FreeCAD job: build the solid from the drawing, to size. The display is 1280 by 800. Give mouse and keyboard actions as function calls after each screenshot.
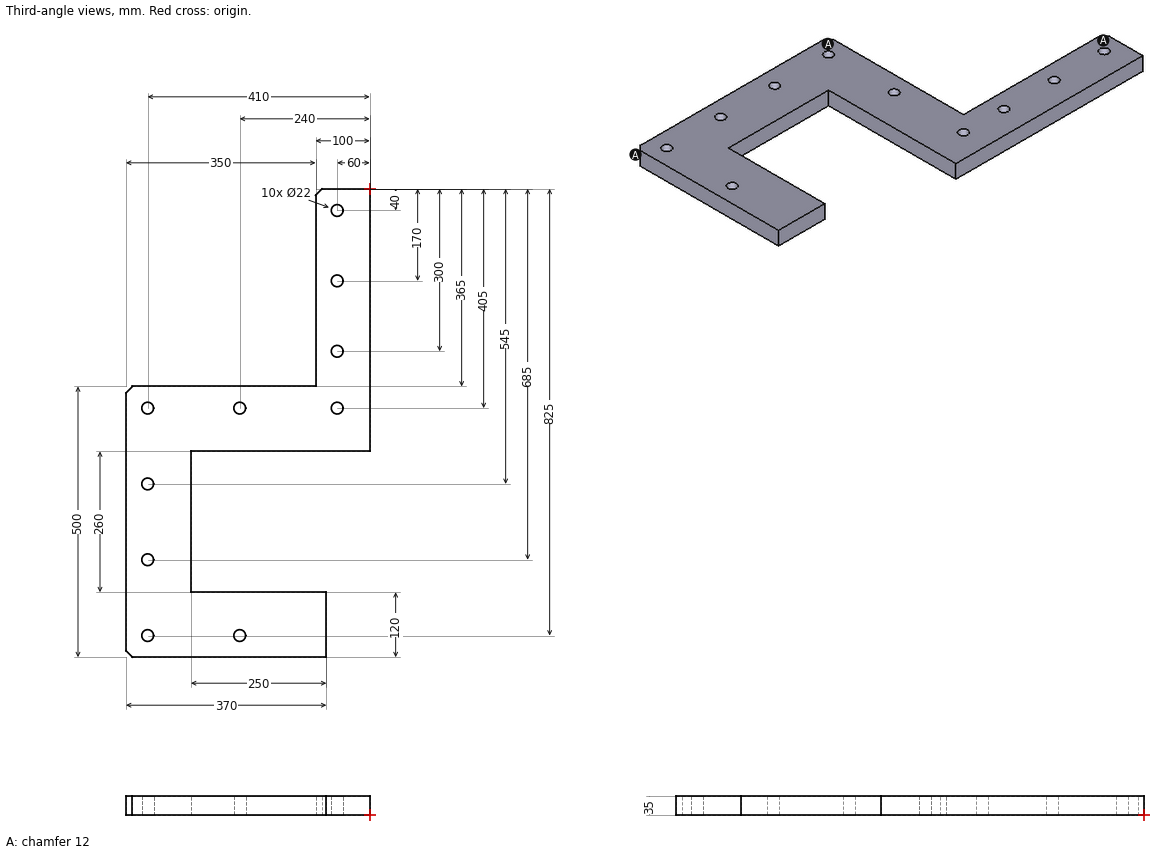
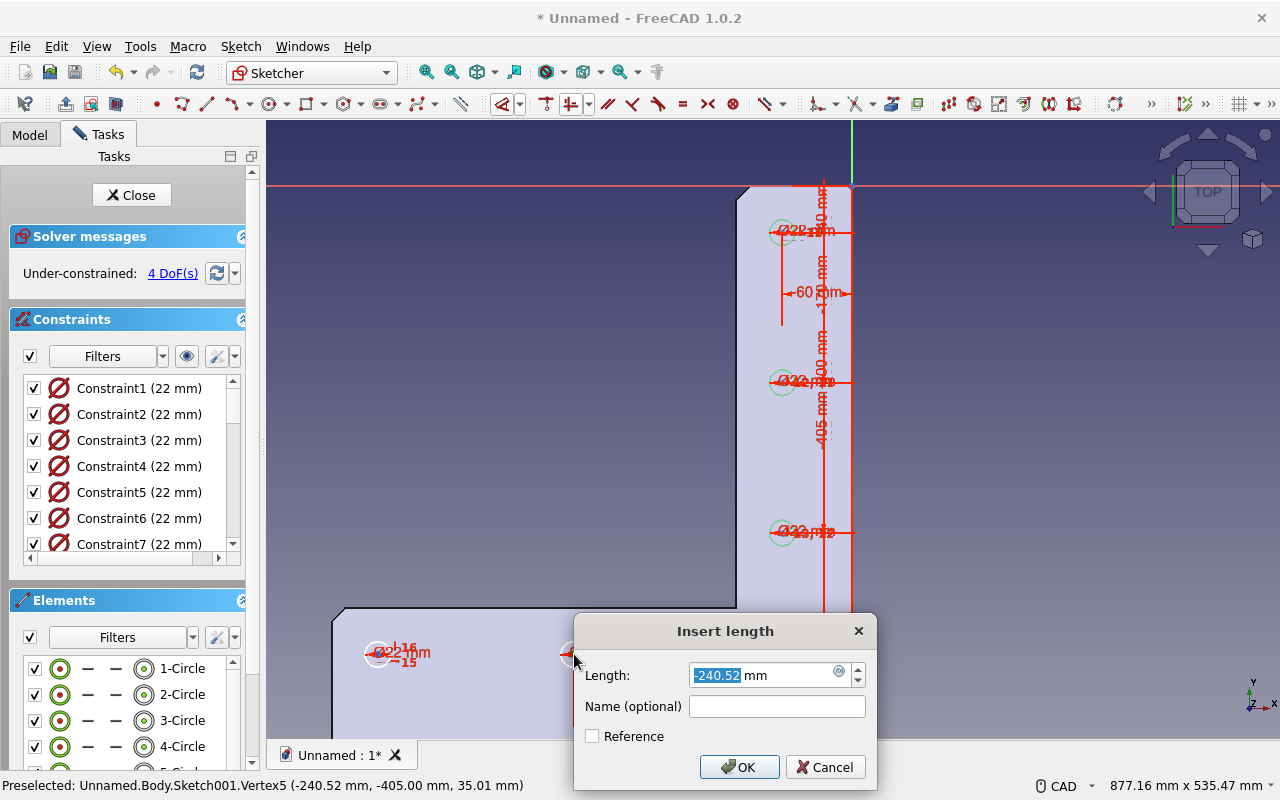
text(-240)
key(Return)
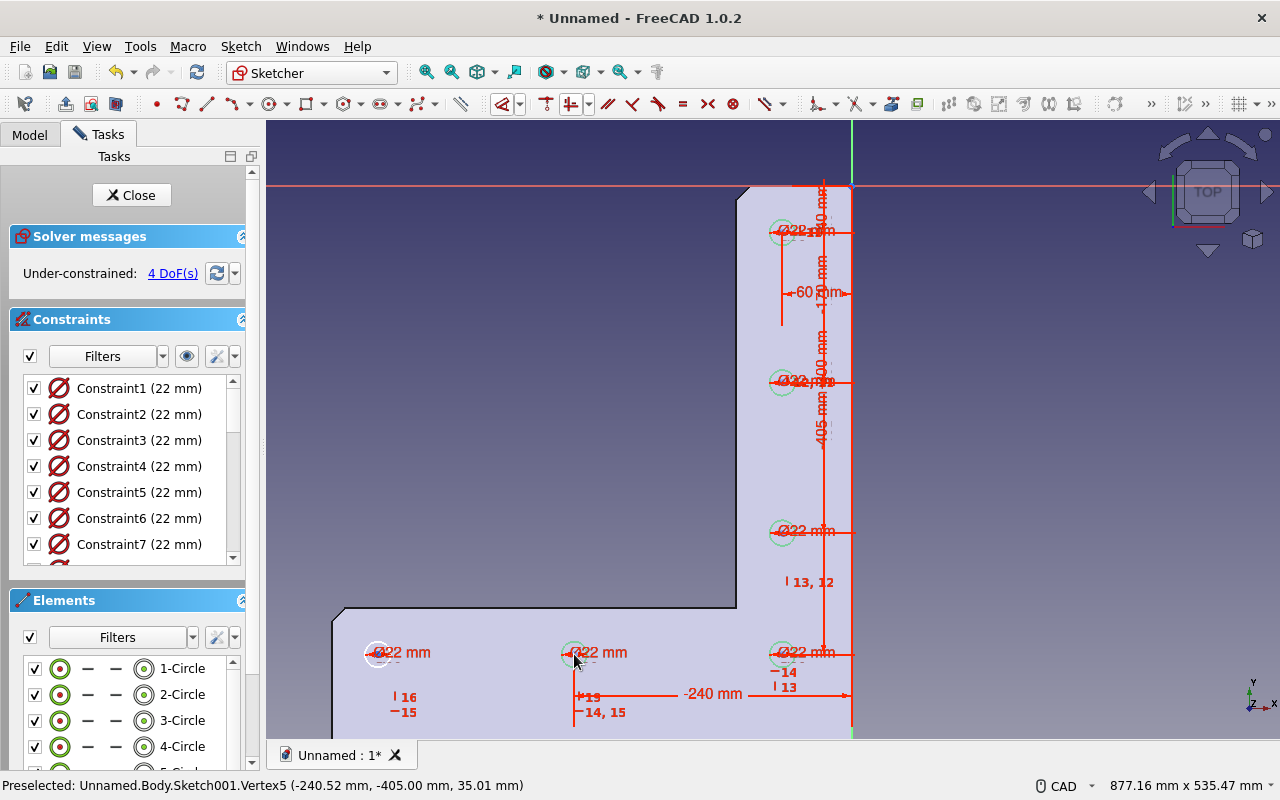
click(378, 654)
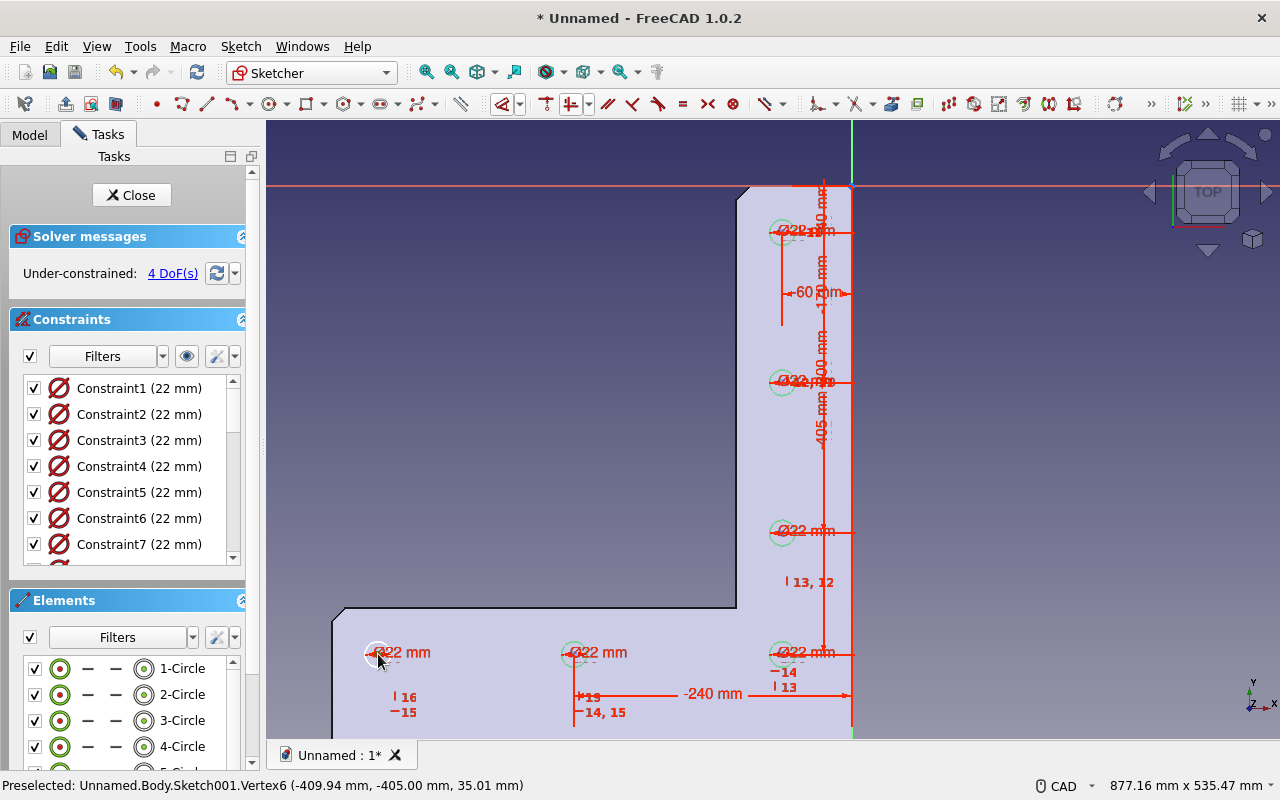
key(l)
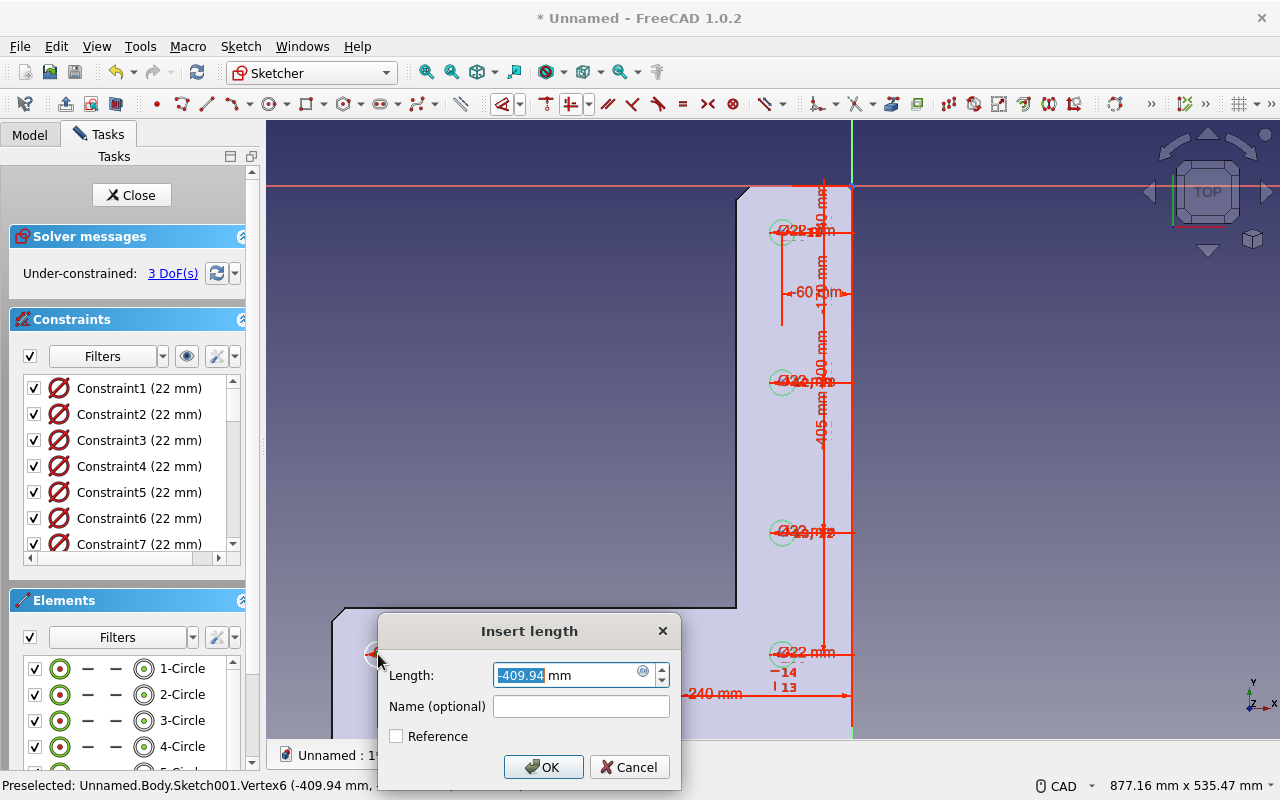
text(-410)
key(Return)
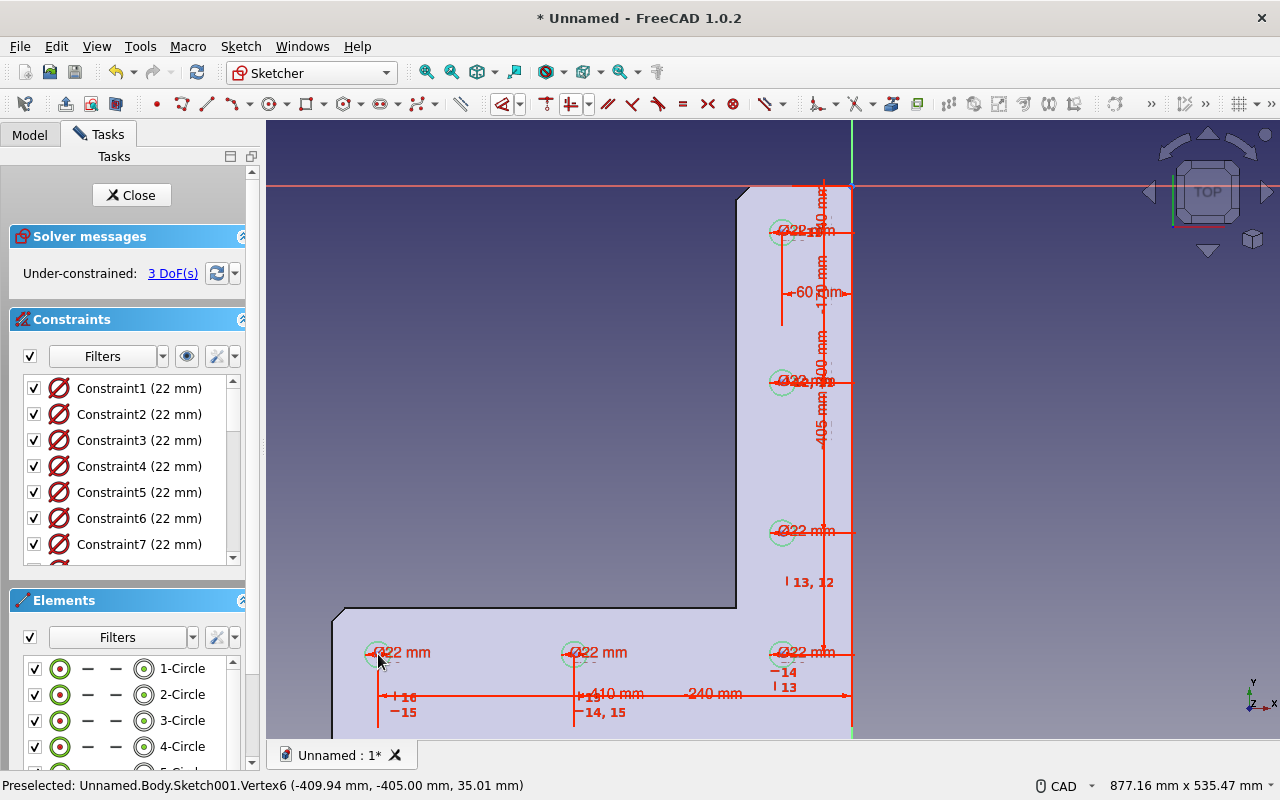
scroll(783, 234, down, 4)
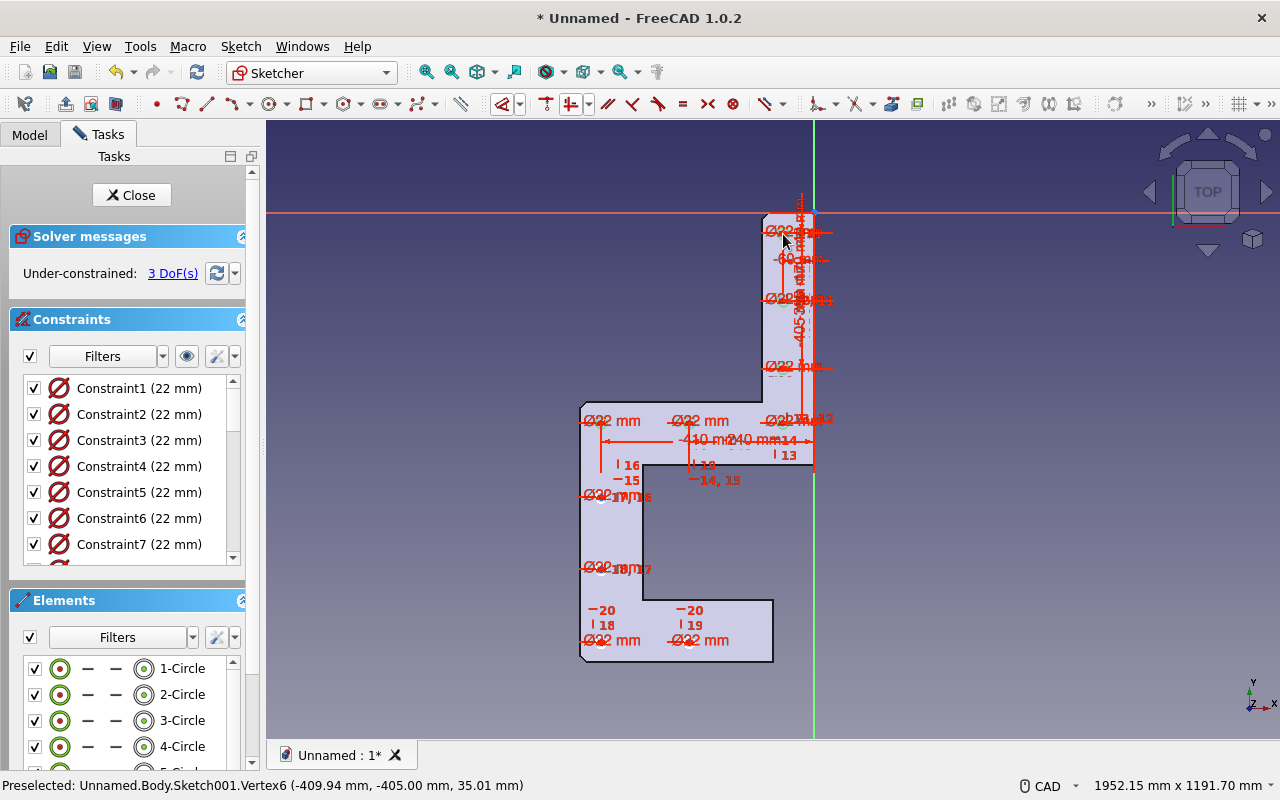
click(601, 497)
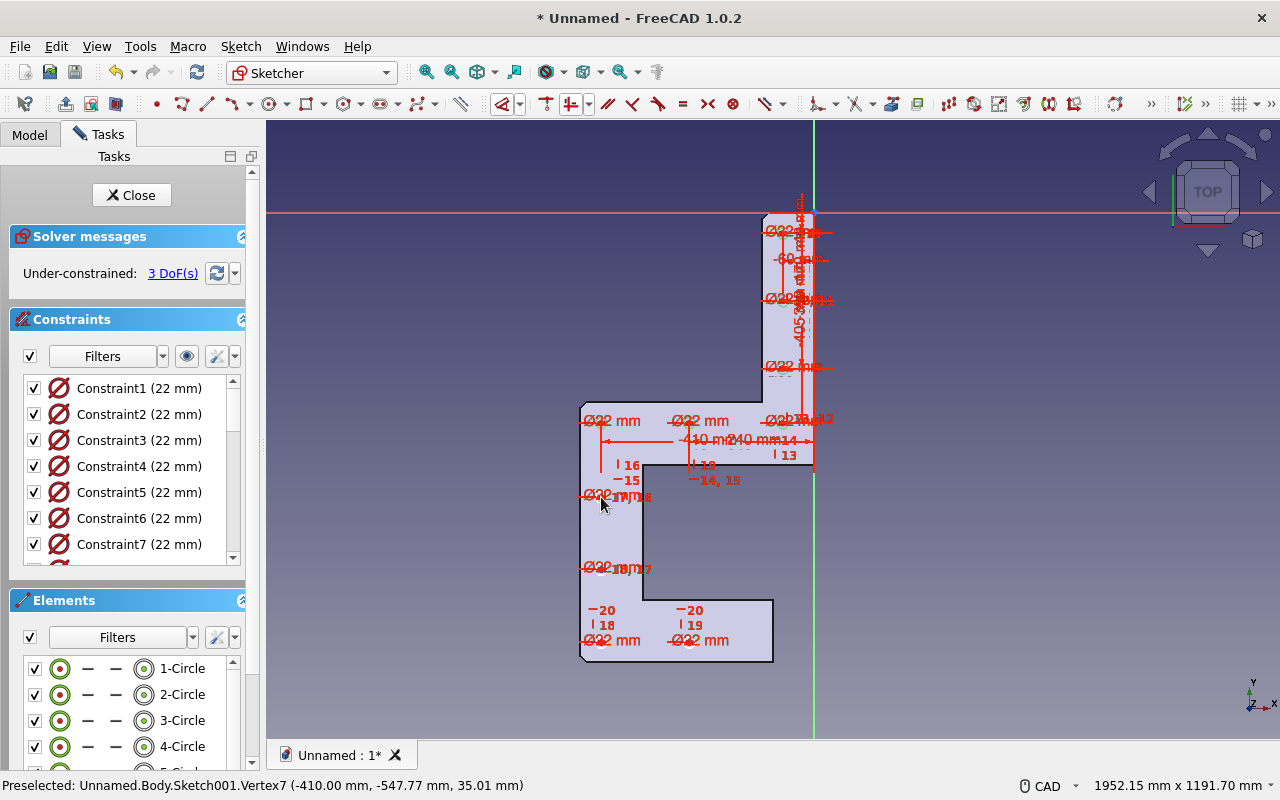
click(520, 104)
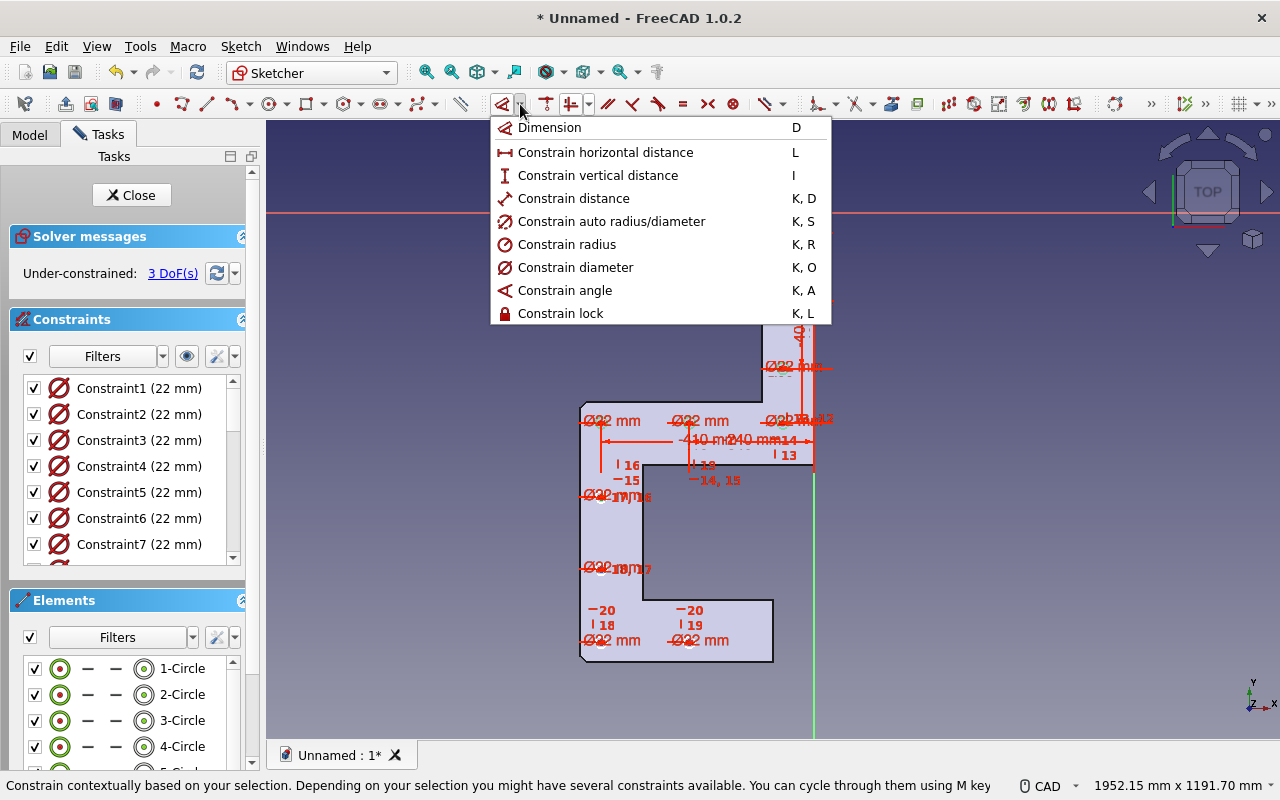
click(661, 176)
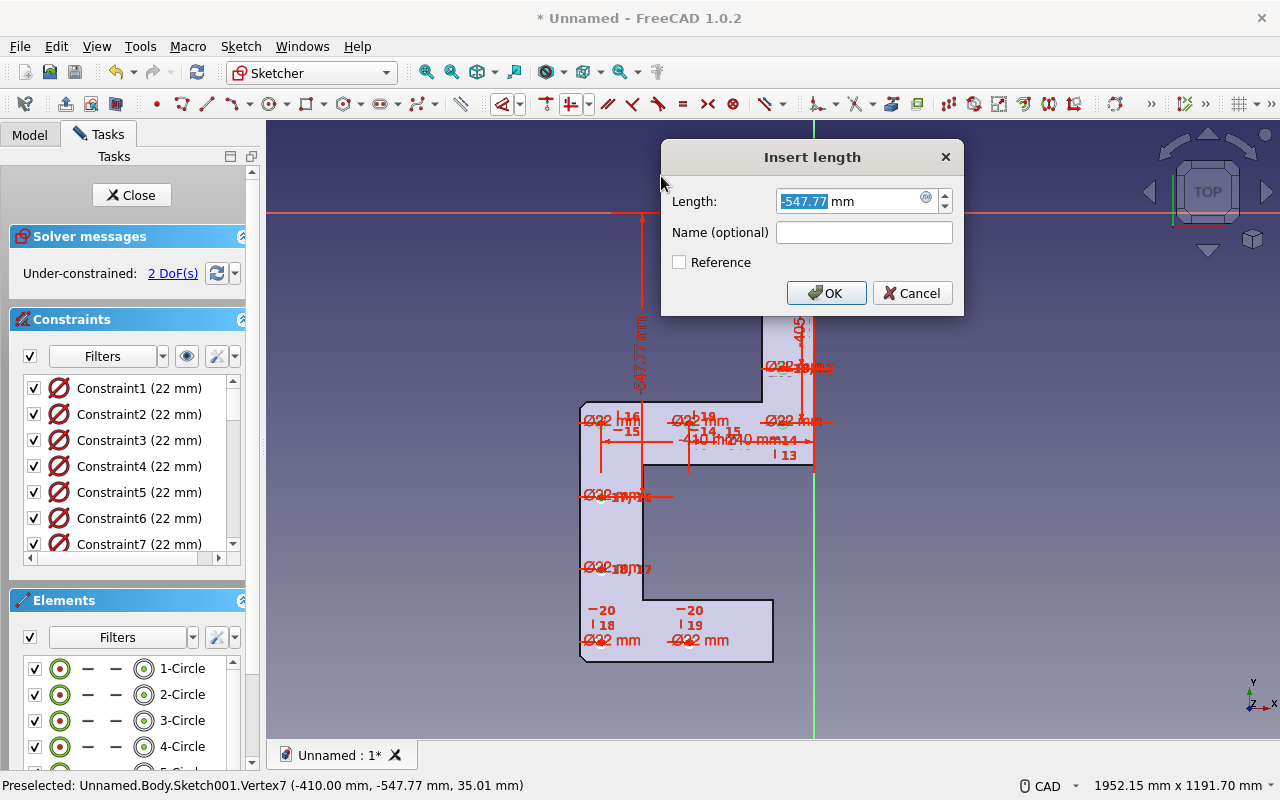
text(-545)
key(Return)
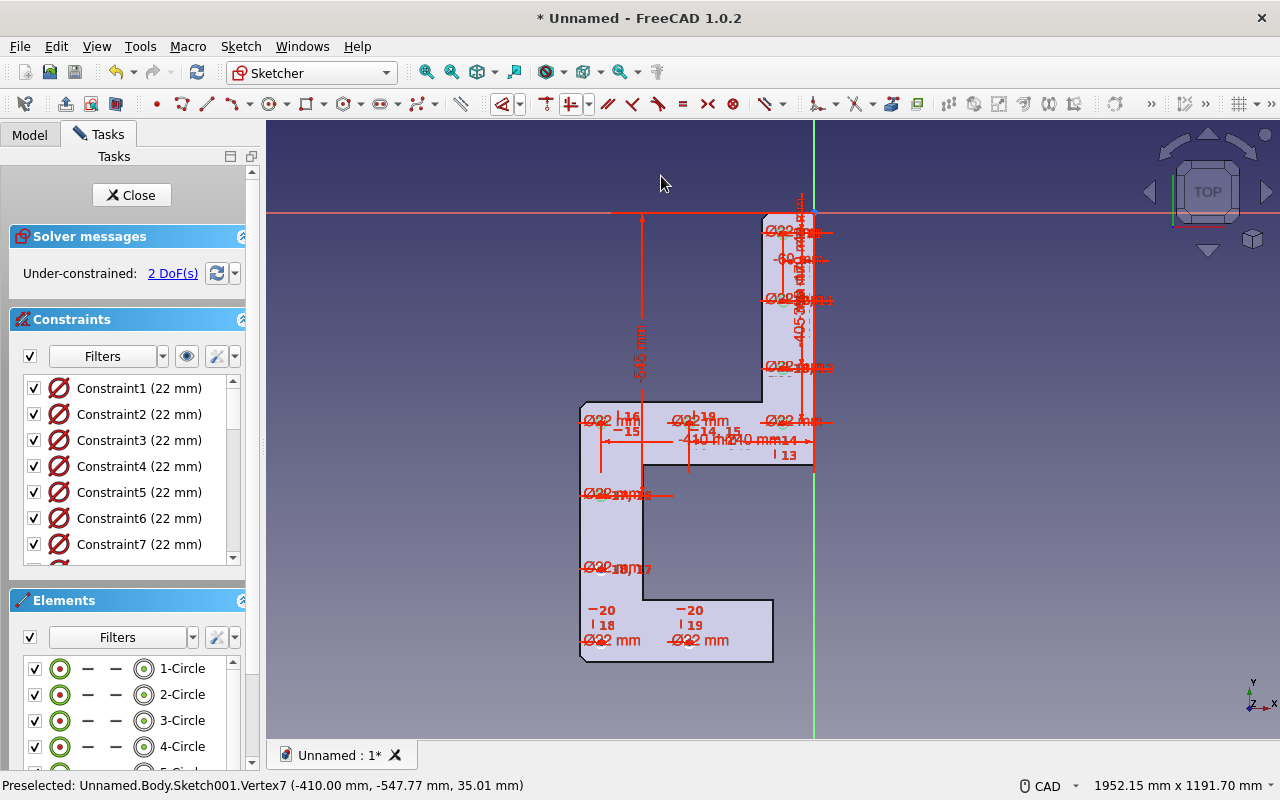
click(601, 569)